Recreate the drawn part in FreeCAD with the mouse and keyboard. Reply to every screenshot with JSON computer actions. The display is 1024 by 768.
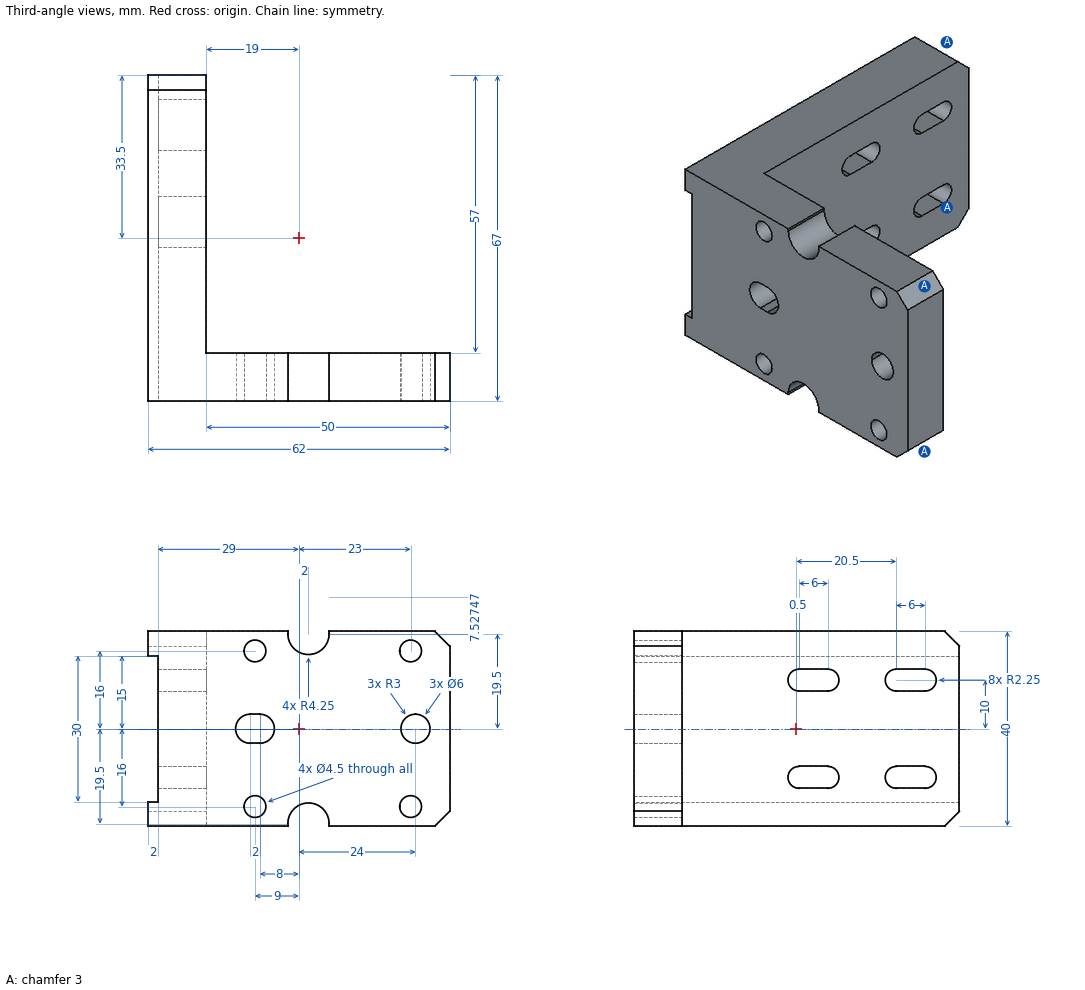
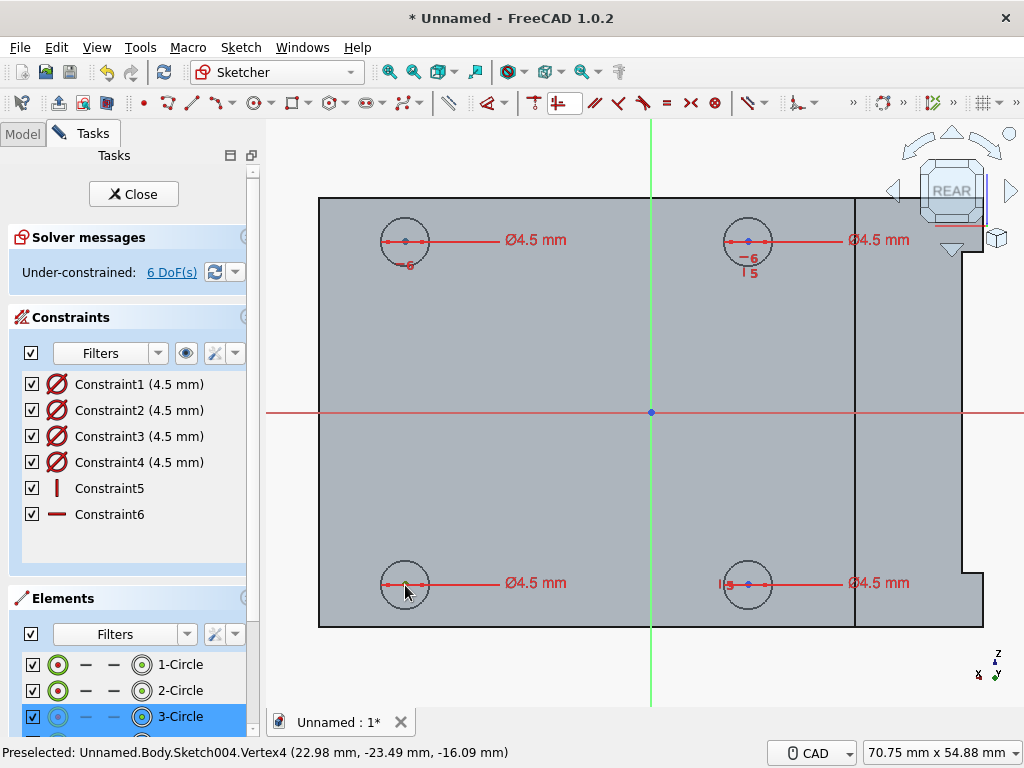
{"action": "key", "text": "v"}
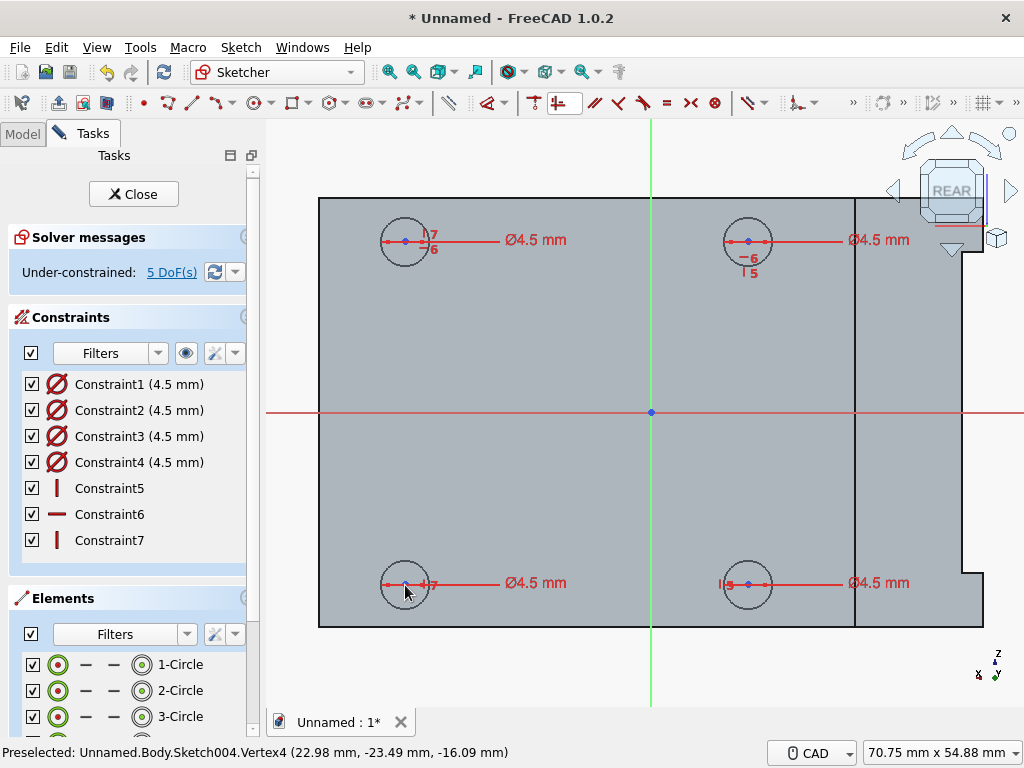
{"action": "left_click", "coordinate": [748, 585]}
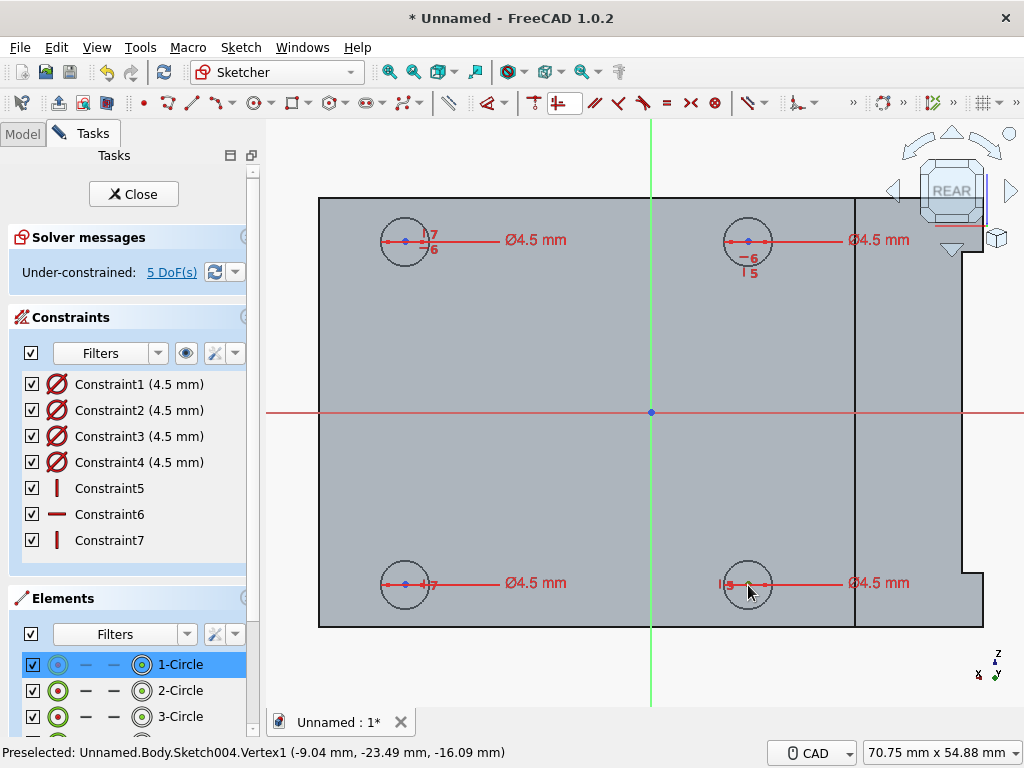
{"action": "left_click", "coordinate": [405, 585]}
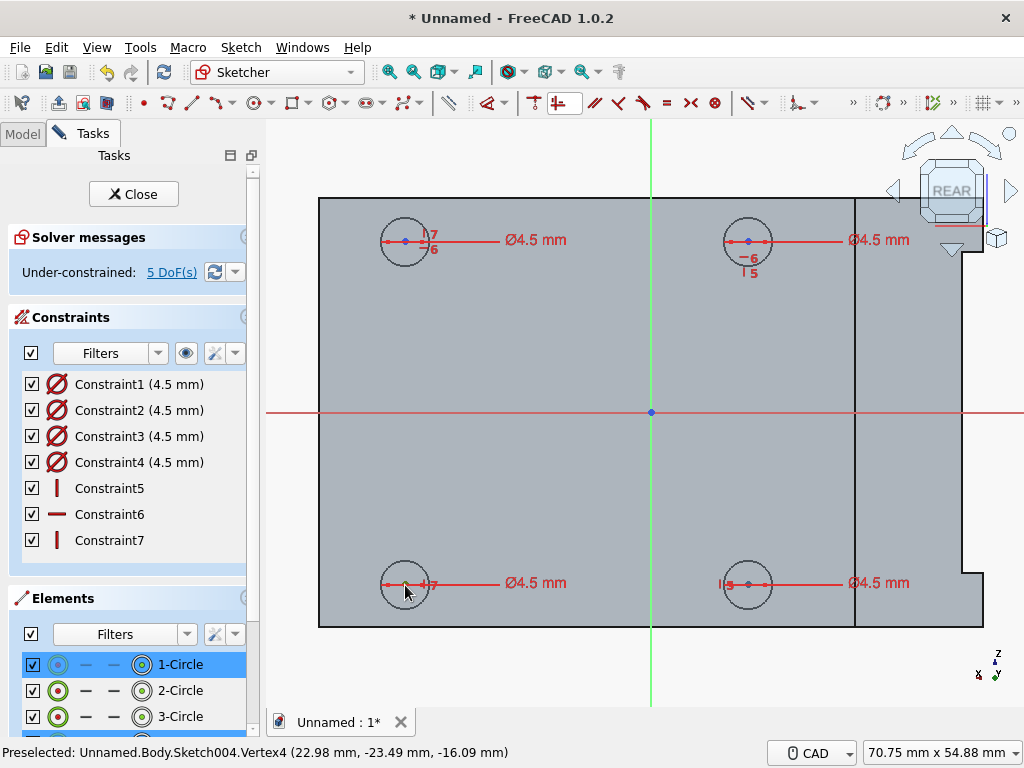
{"action": "left_click", "coordinate": [576, 104]}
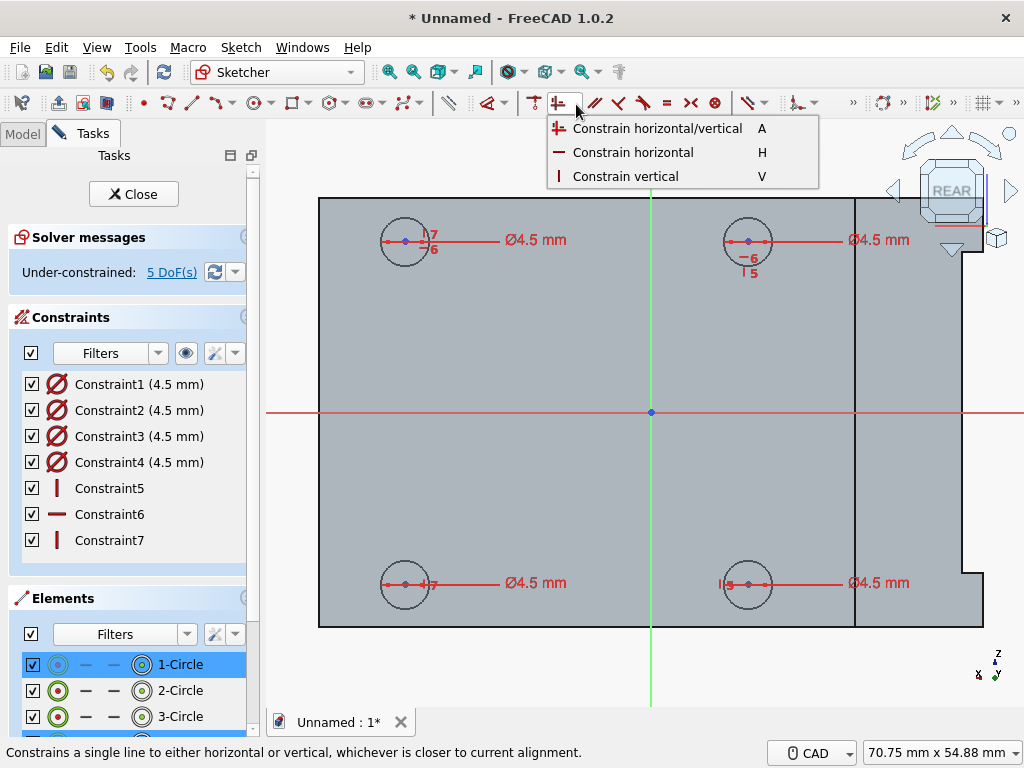
{"action": "left_click", "coordinate": [683, 152]}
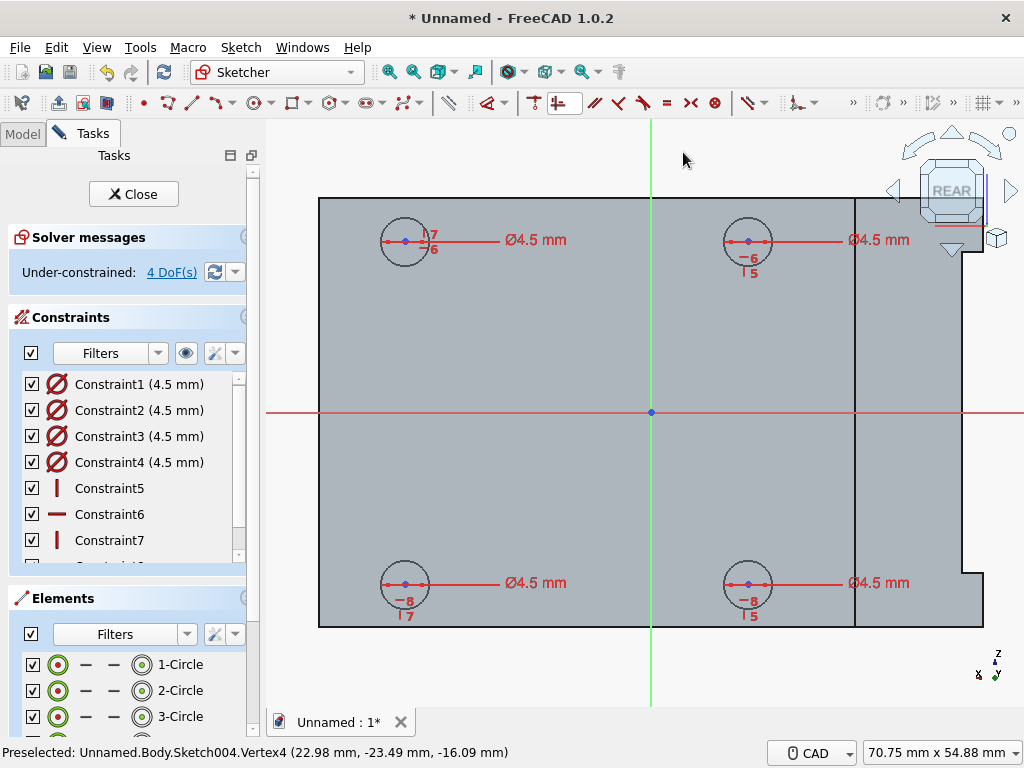
{"action": "left_click", "coordinate": [488, 104]}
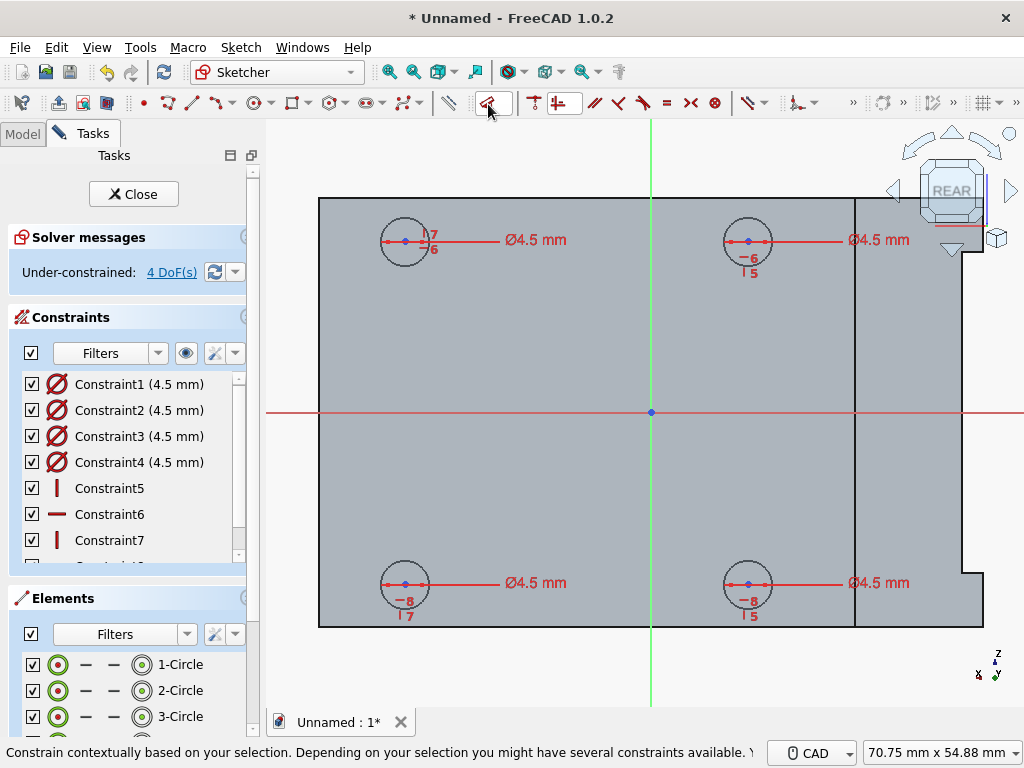
{"action": "left_click", "coordinate": [748, 585]}
{"action": "left_click", "coordinate": [700, 619]}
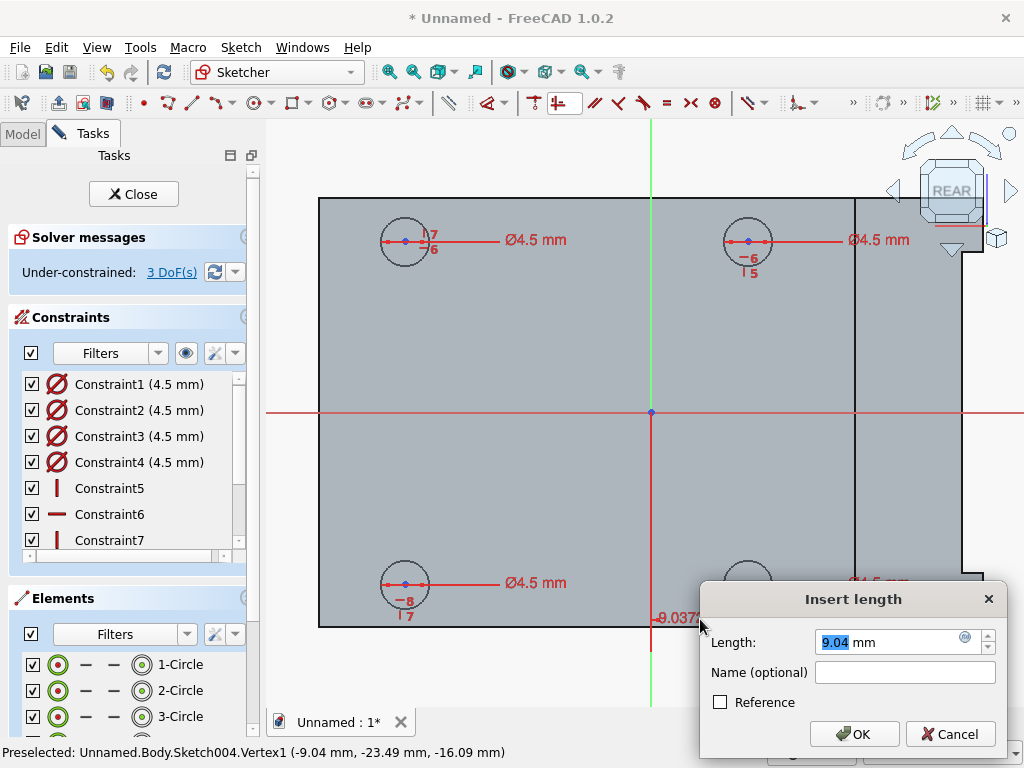
{"action": "type", "text": "9"}
{"action": "key", "text": "Return"}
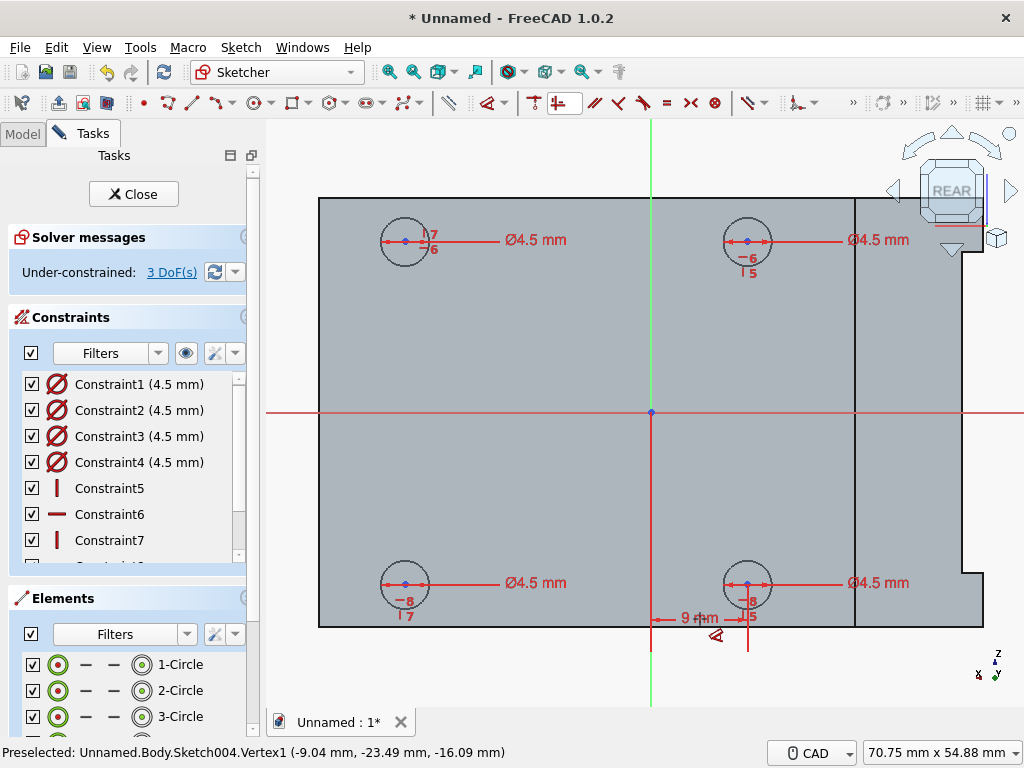
{"action": "left_click", "coordinate": [748, 585]}
{"action": "left_click", "coordinate": [782, 499]}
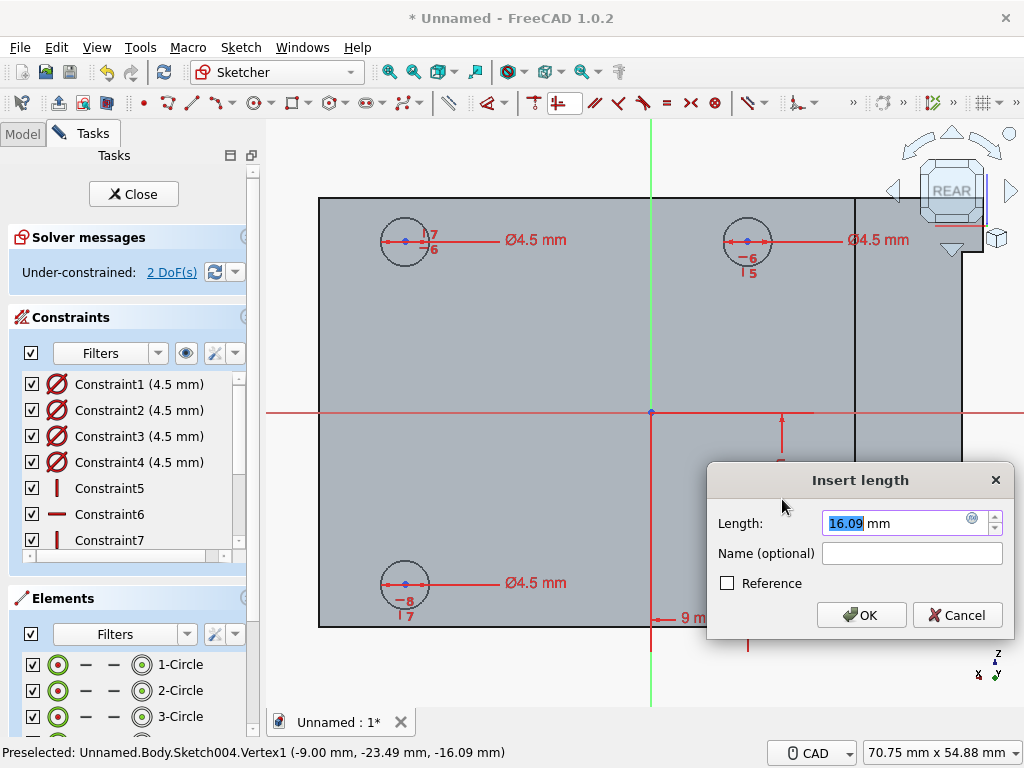
{"action": "type", "text": "16"}
{"action": "key", "text": "Return"}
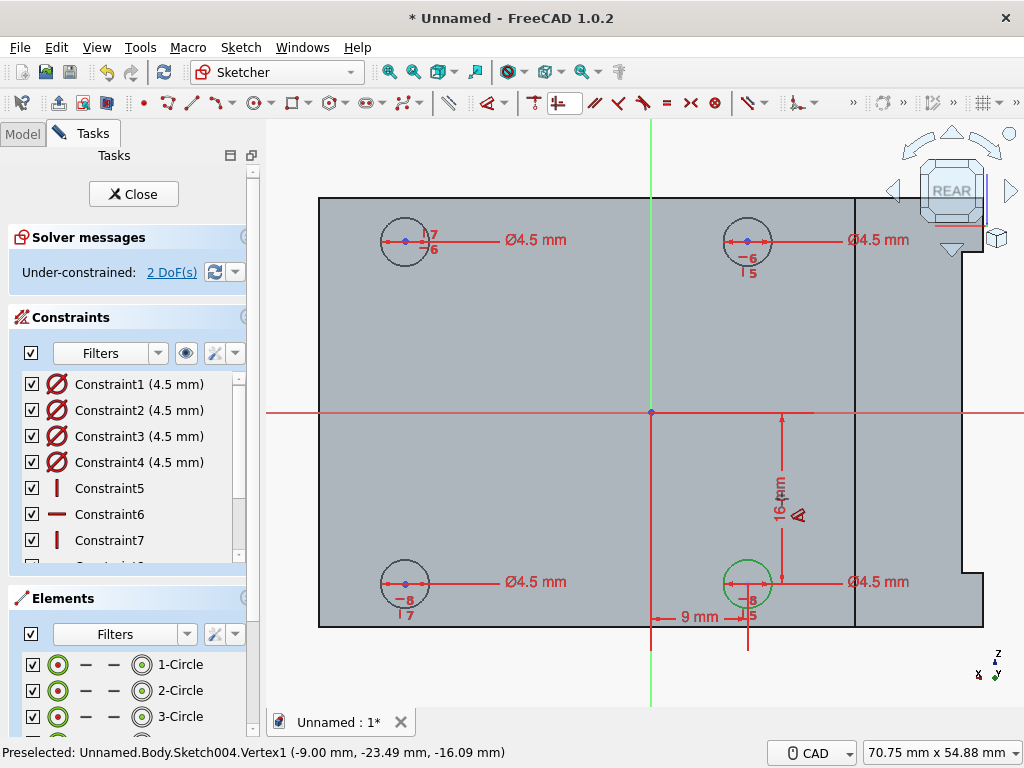
{"action": "left_click", "coordinate": [748, 242]}
{"action": "left_click", "coordinate": [782, 327]}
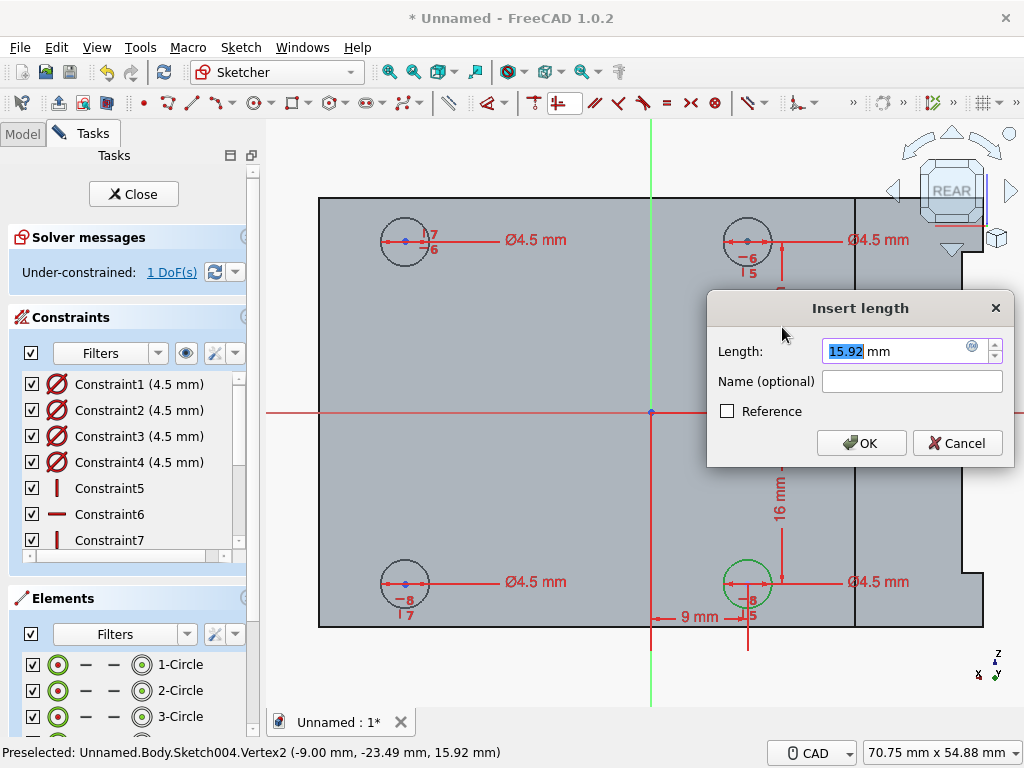
{"action": "type", "text": "16"}
{"action": "key", "text": "Return"}